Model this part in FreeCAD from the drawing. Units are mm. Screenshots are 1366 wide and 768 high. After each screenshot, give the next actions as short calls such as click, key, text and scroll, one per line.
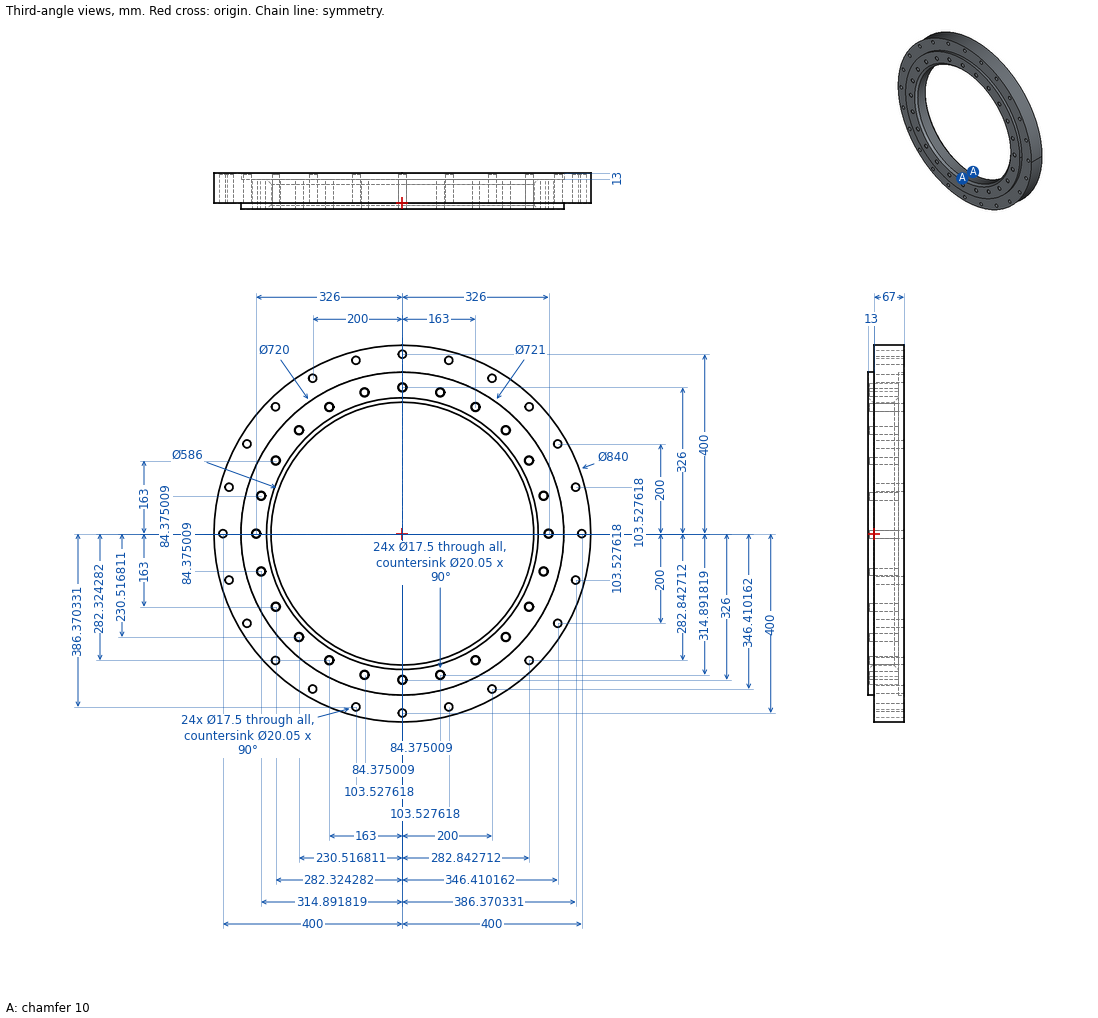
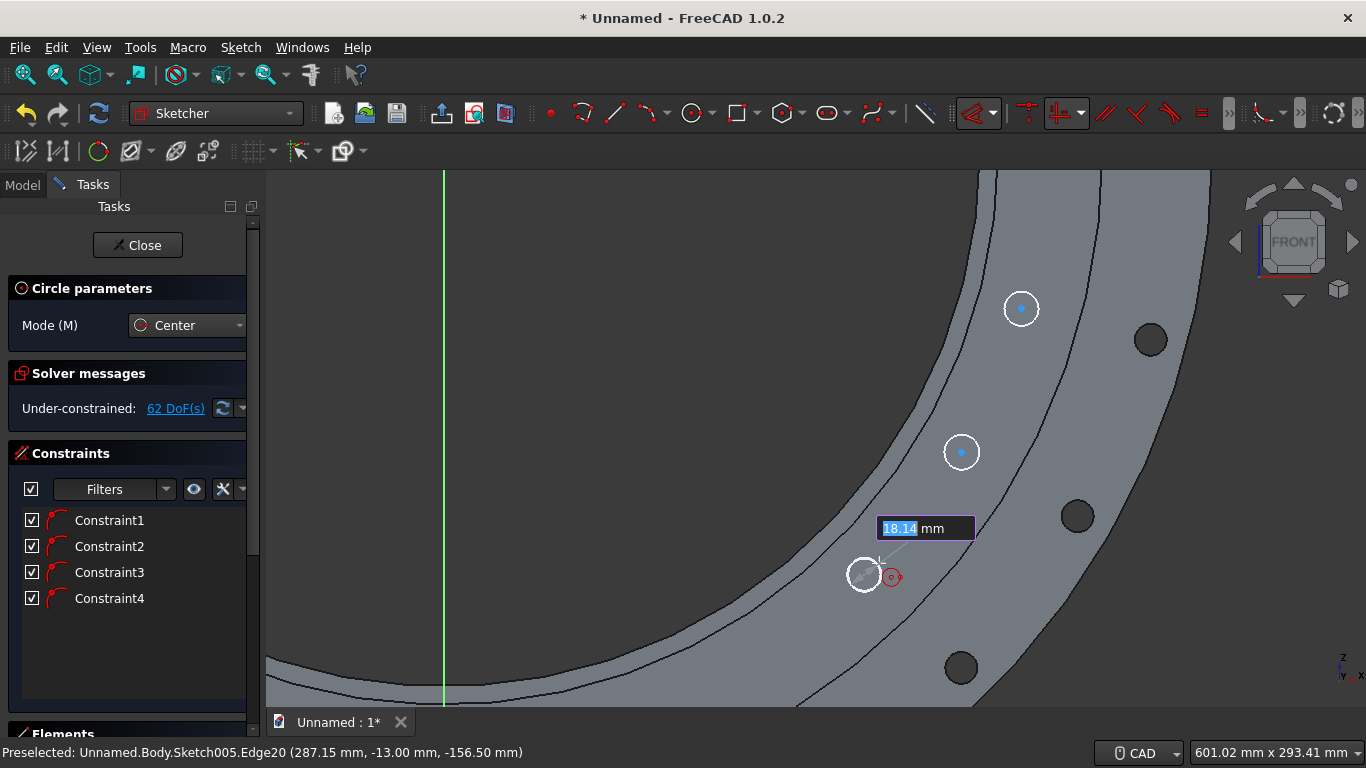
click(877, 561)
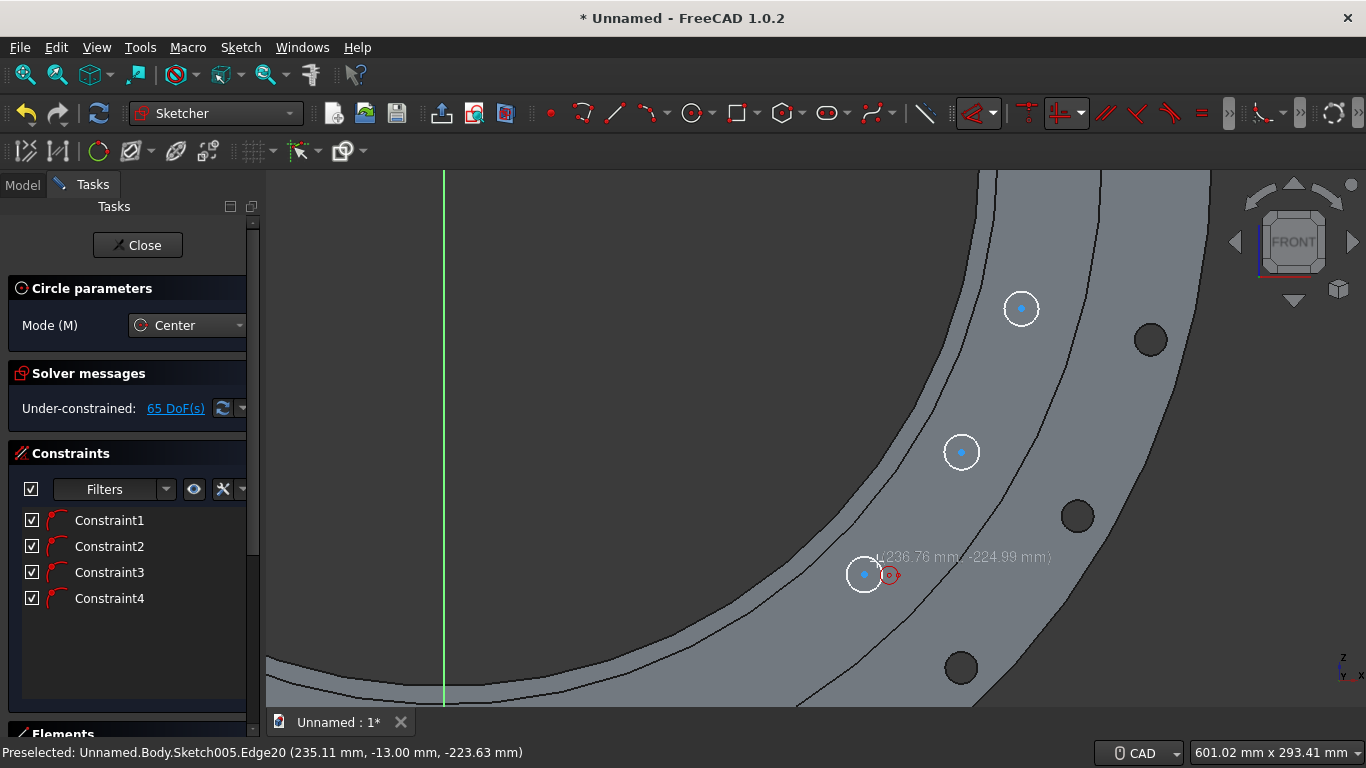
scroll(742, 667, up, 2)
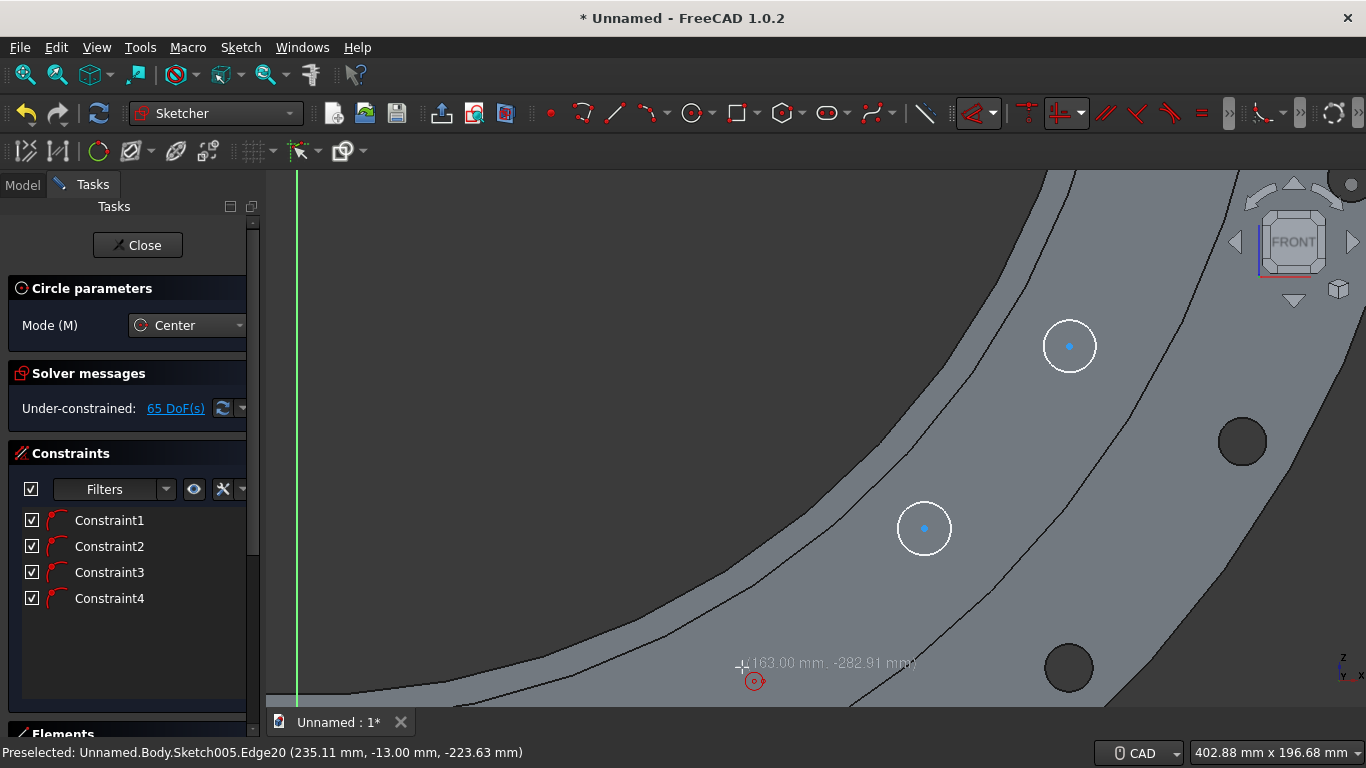
scroll(862, 576, down, 8)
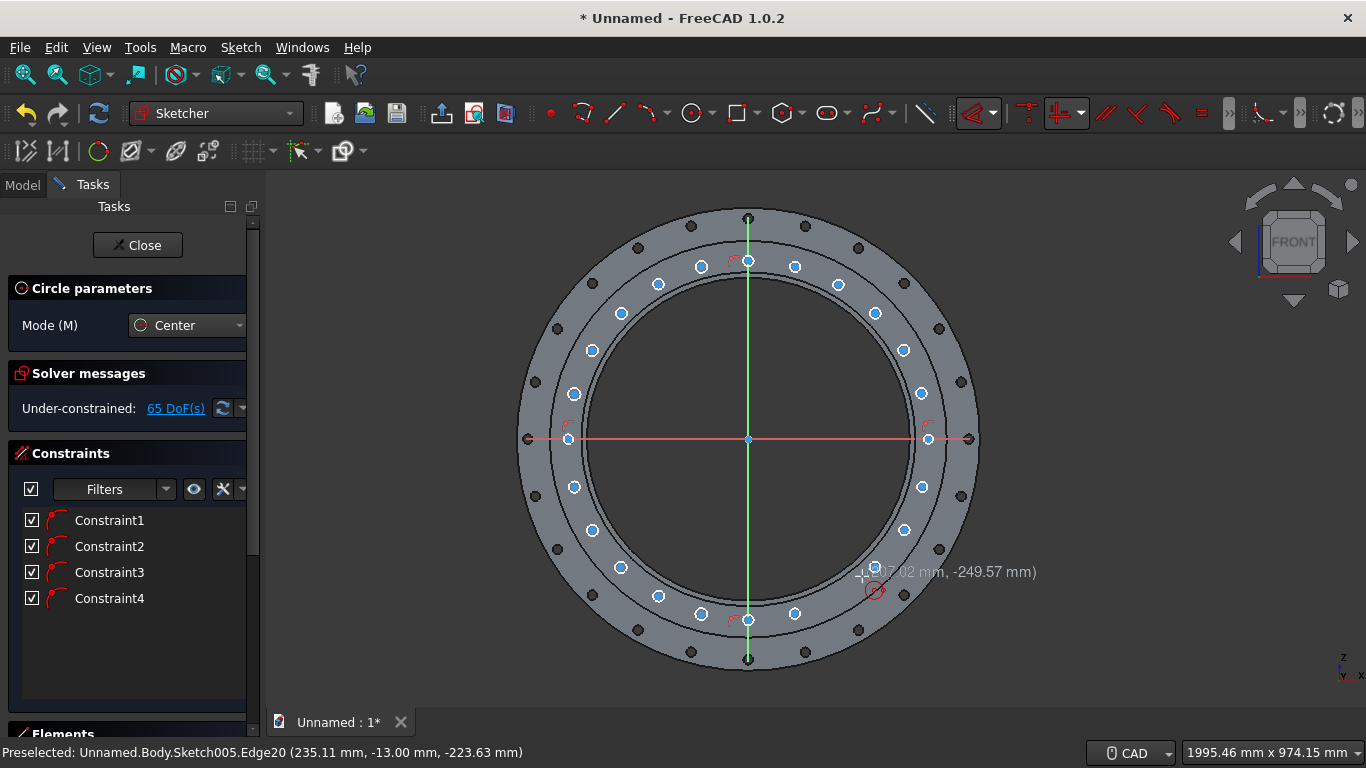
click(838, 595)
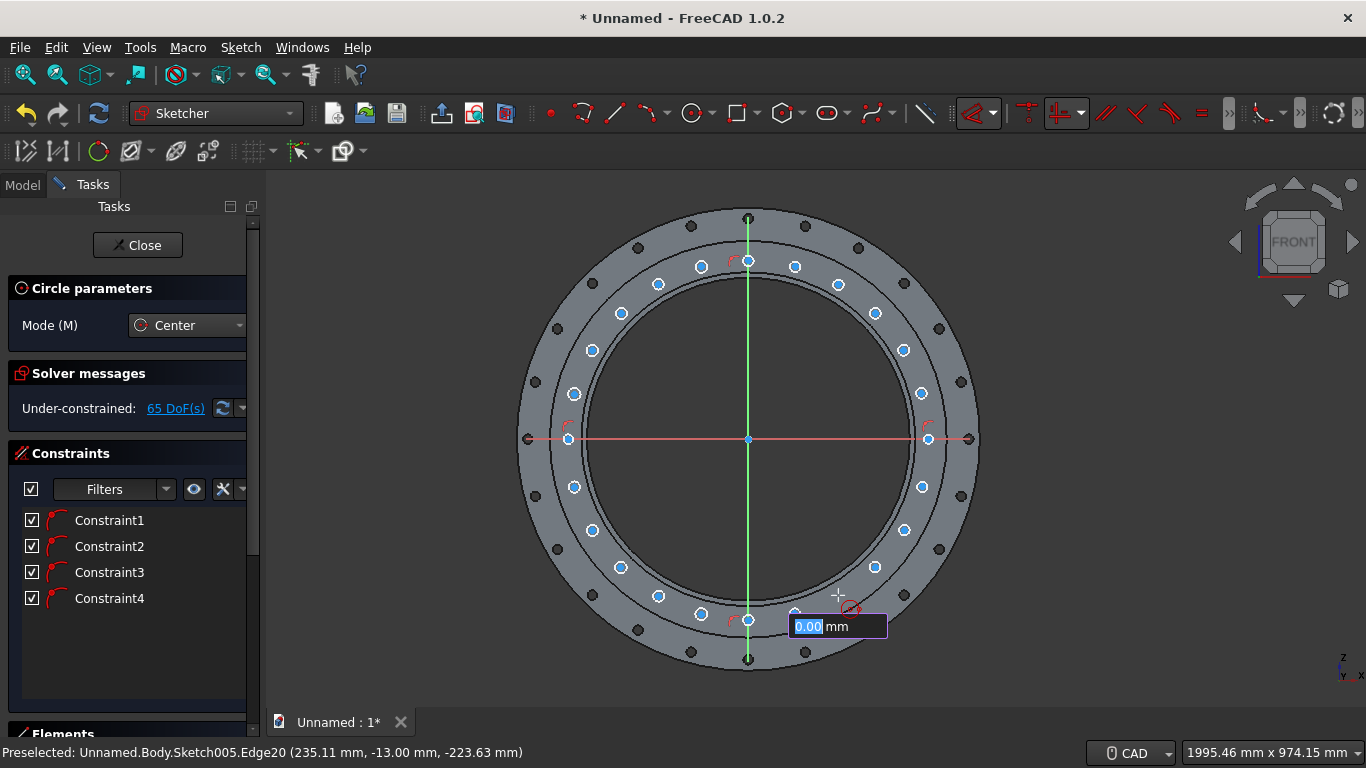
scroll(842, 591, up, 6)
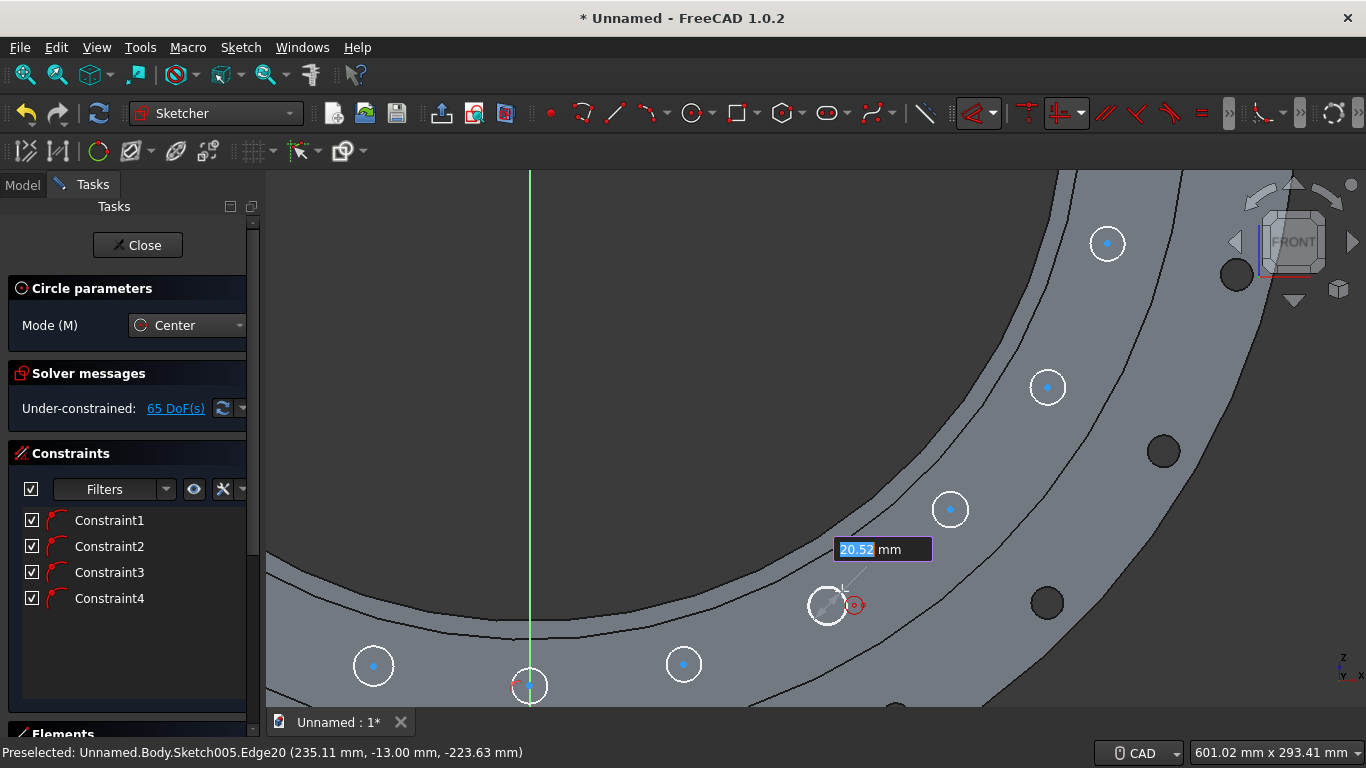
click(839, 591)
key(Escape)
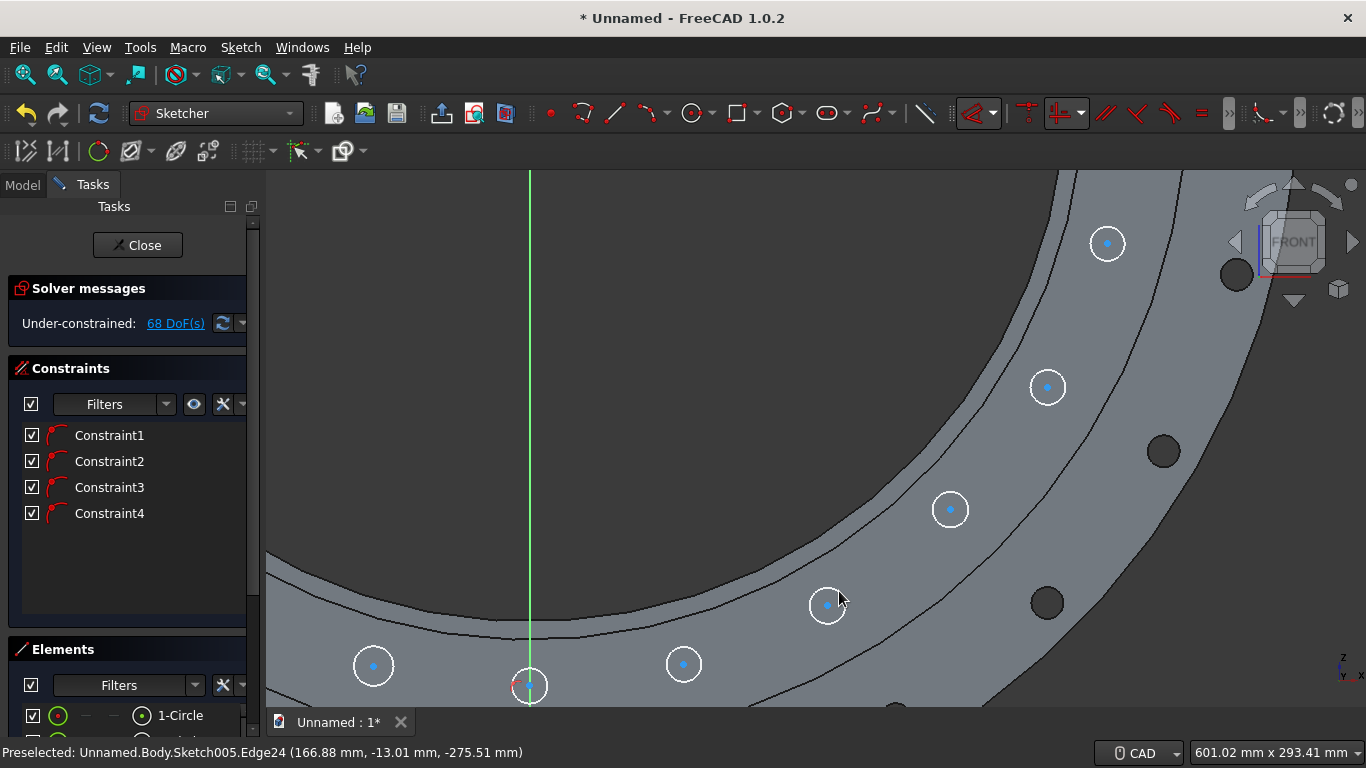
click(696, 652)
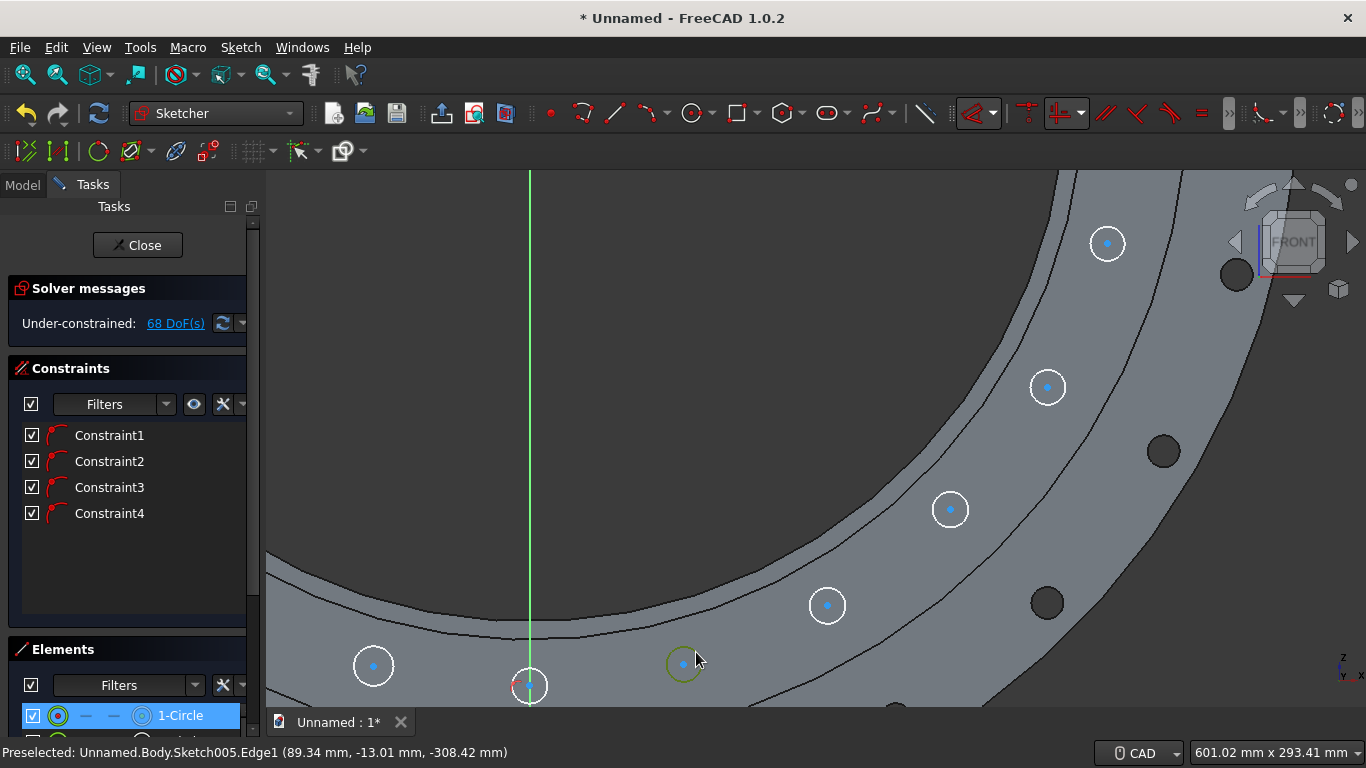
click(542, 673)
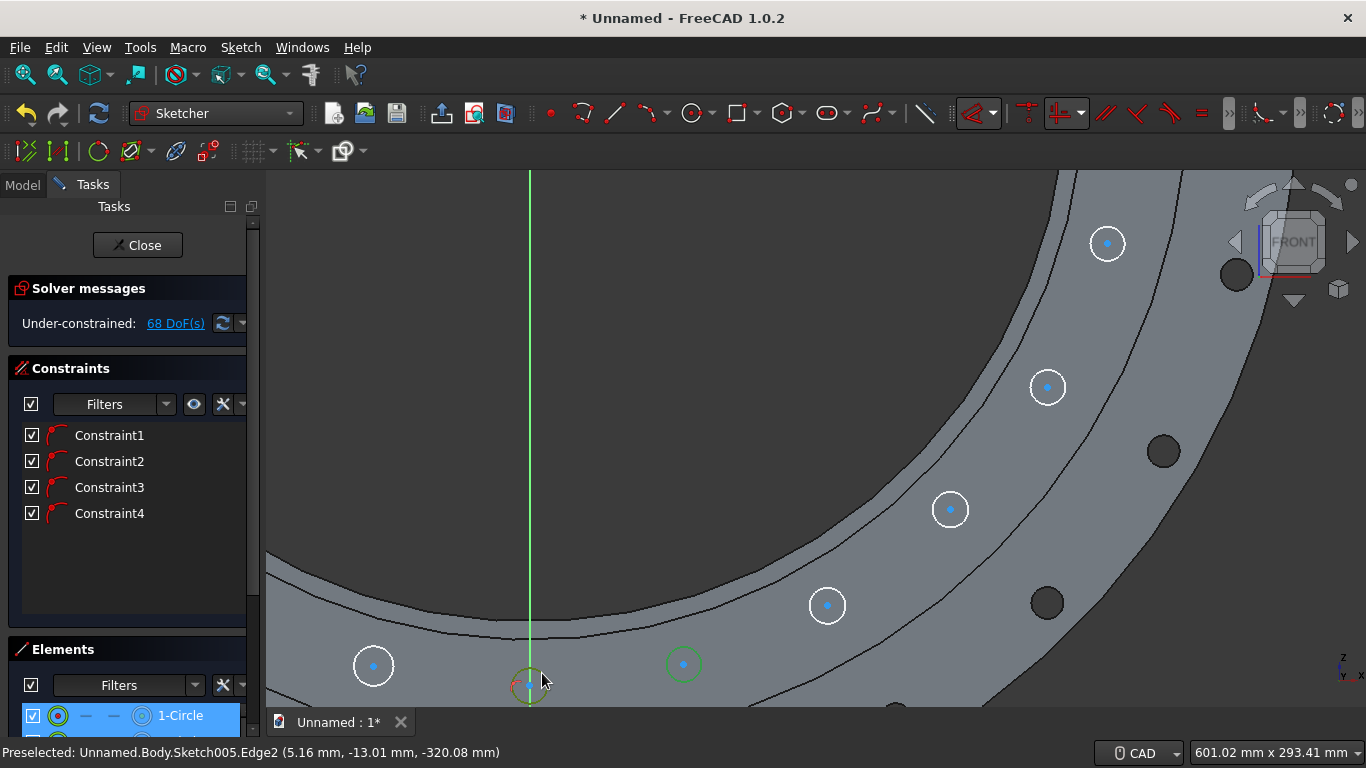
click(388, 652)